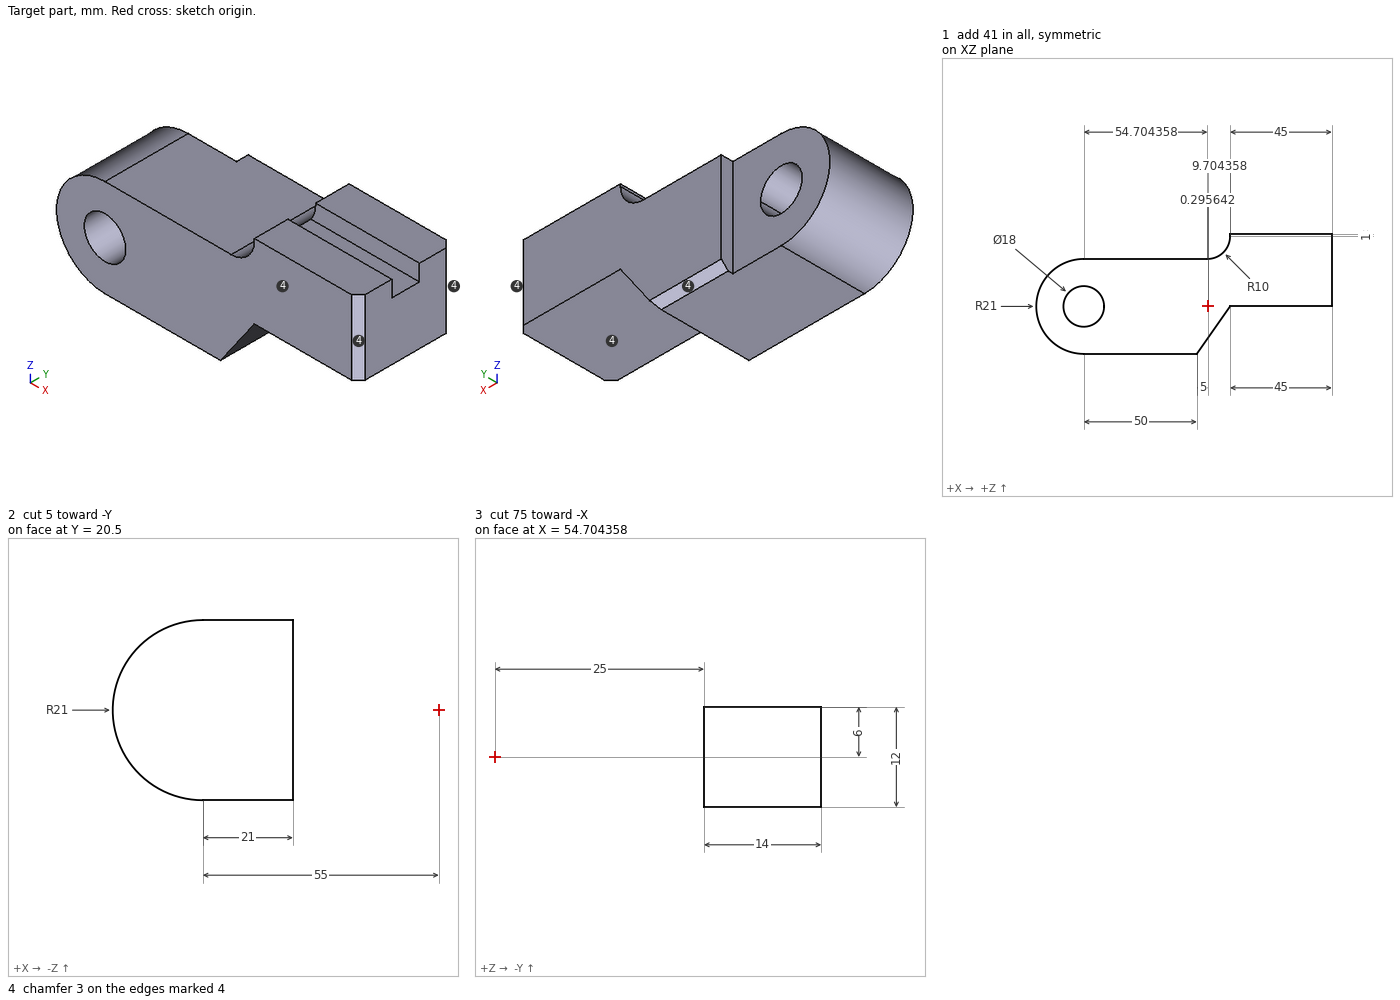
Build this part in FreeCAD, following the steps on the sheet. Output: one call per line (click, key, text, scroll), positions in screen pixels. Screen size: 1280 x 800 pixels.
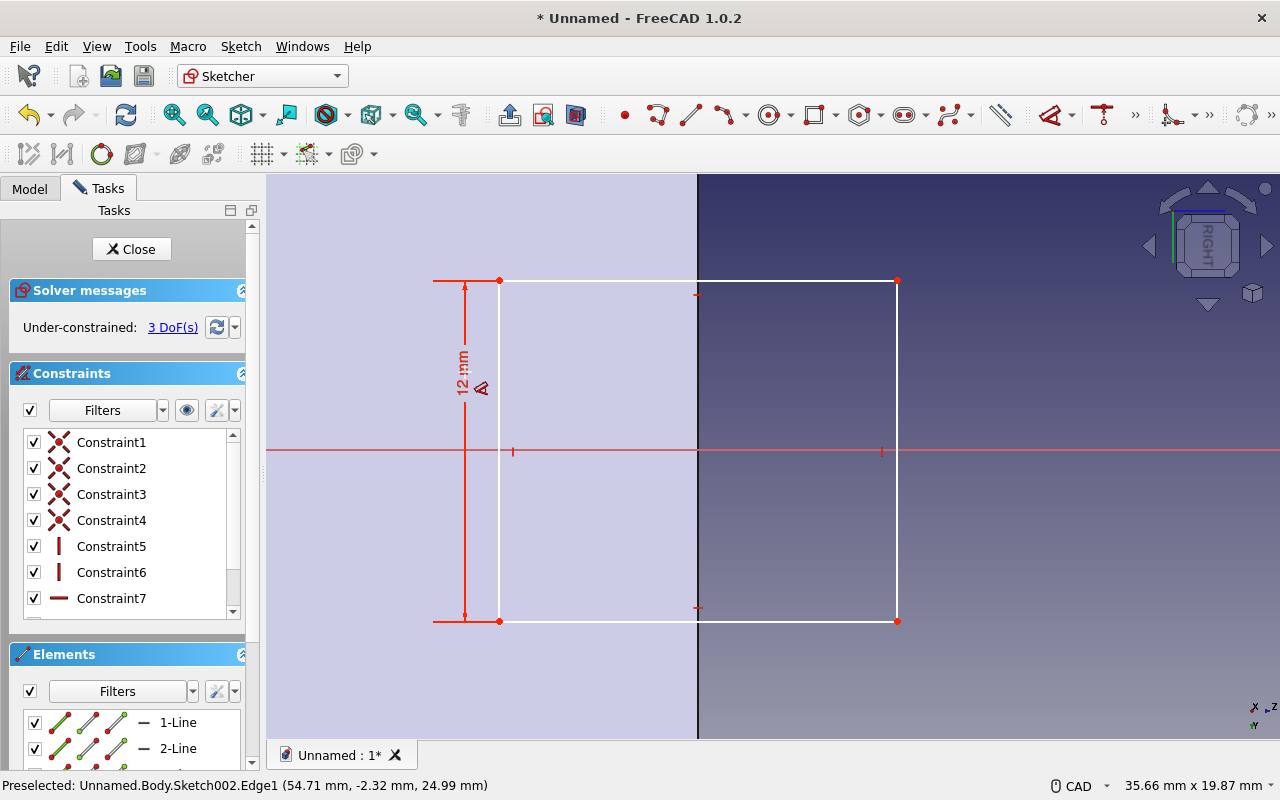
click(618, 622)
click(698, 656)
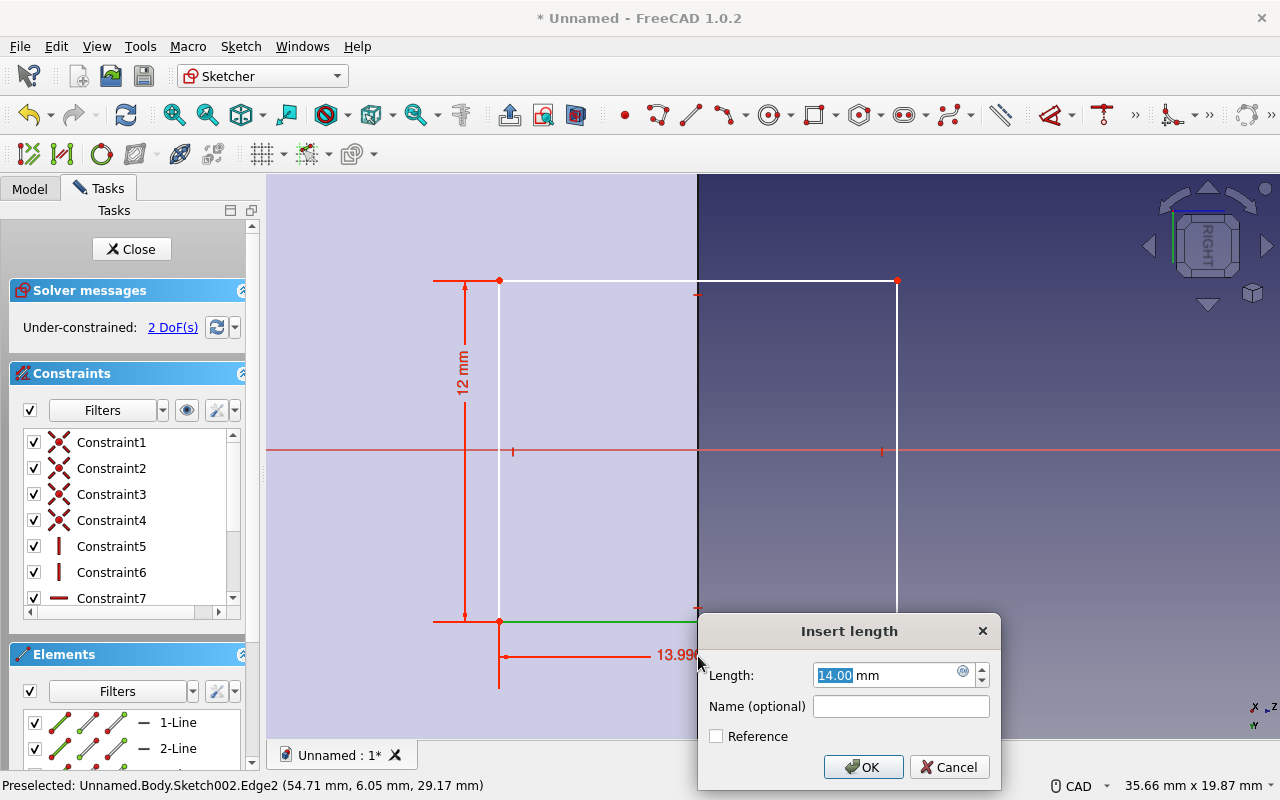
text(14)
key(Return)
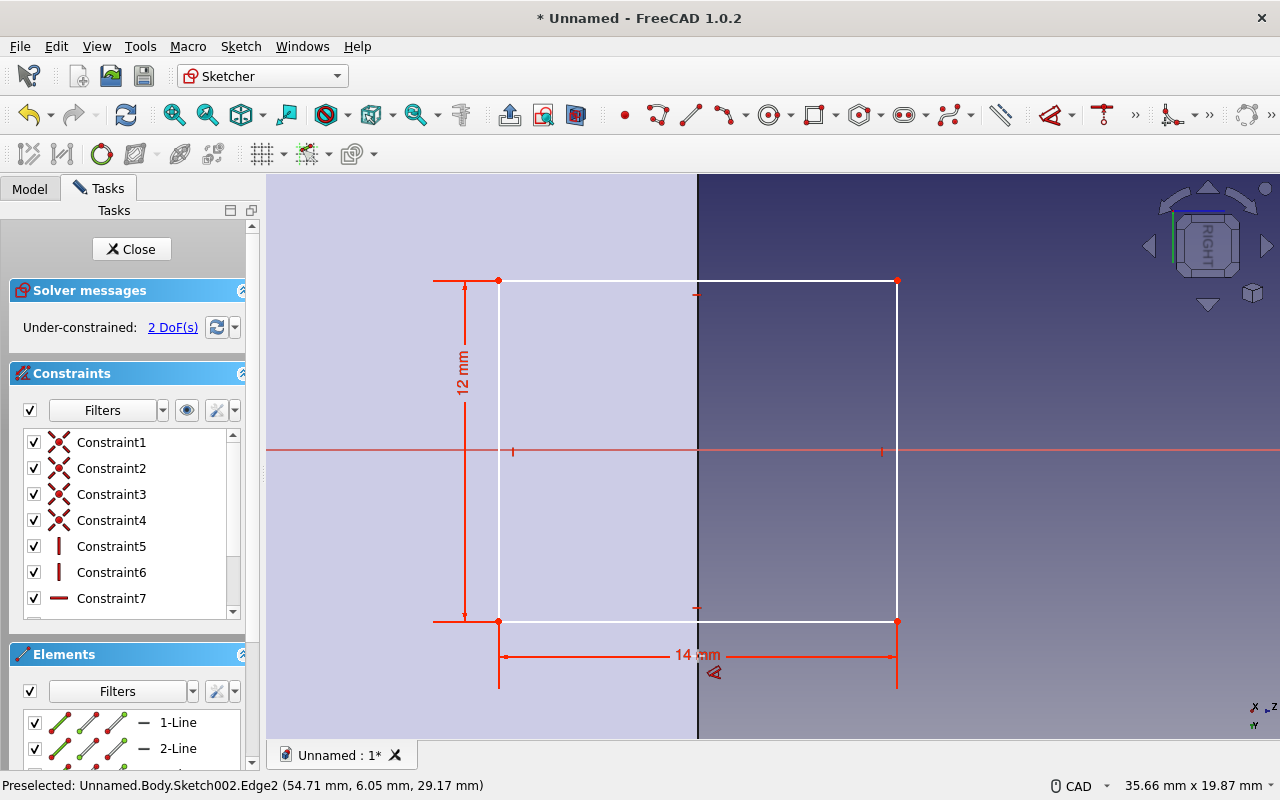
click(499, 281)
click(533, 326)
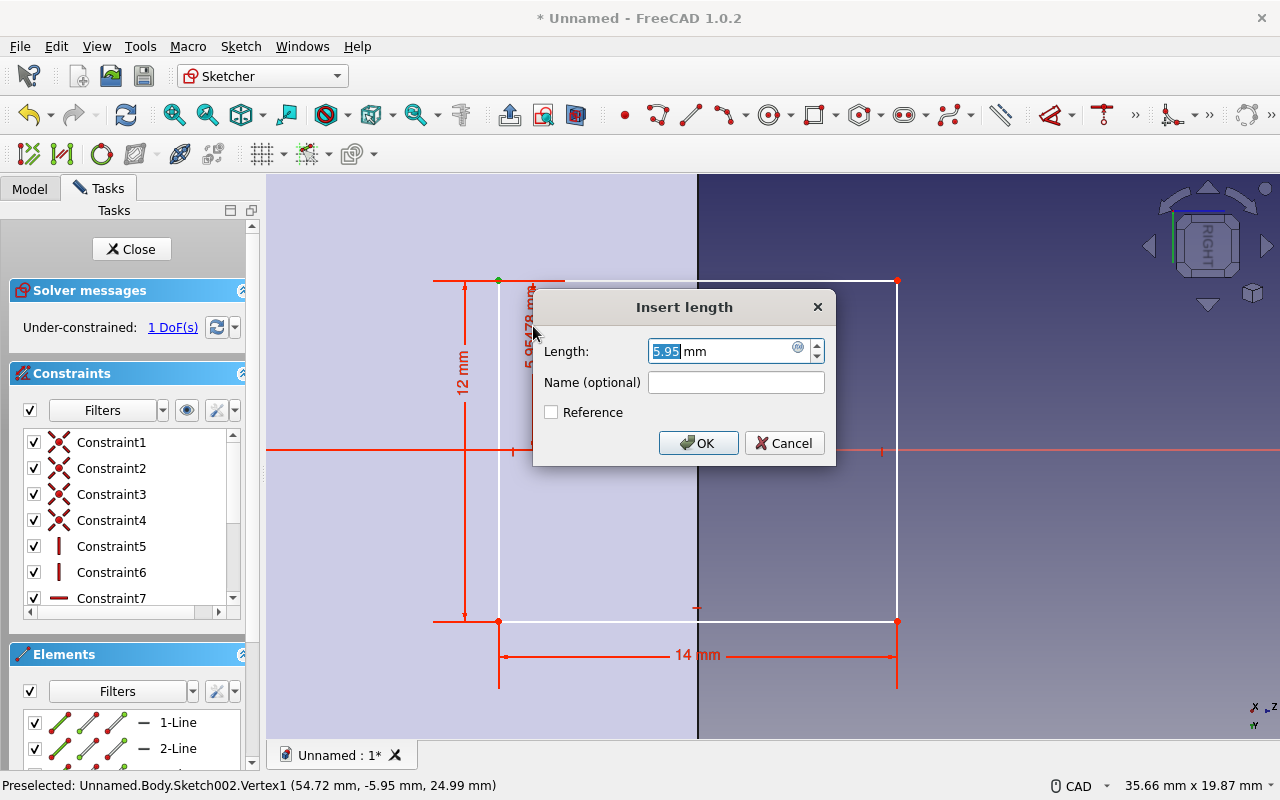
text(6)
key(Return)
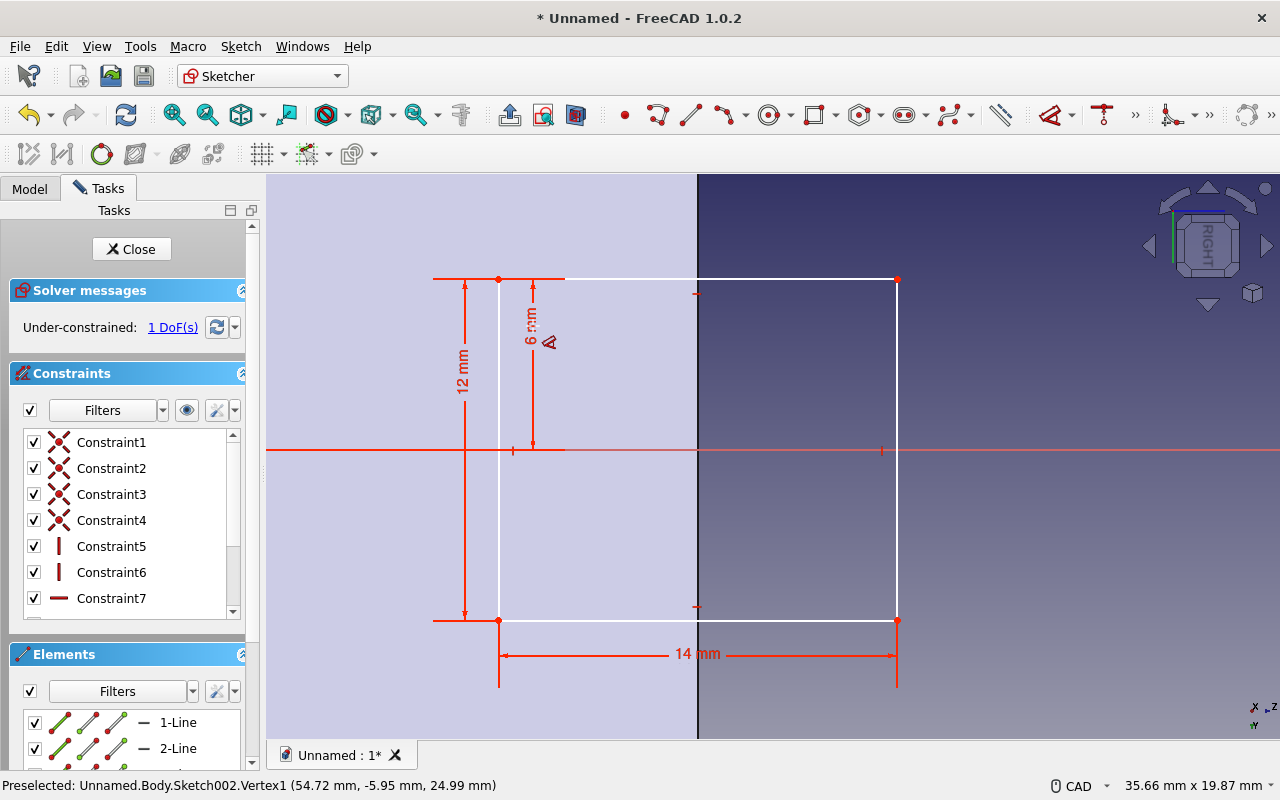
click(499, 279)
click(396, 245)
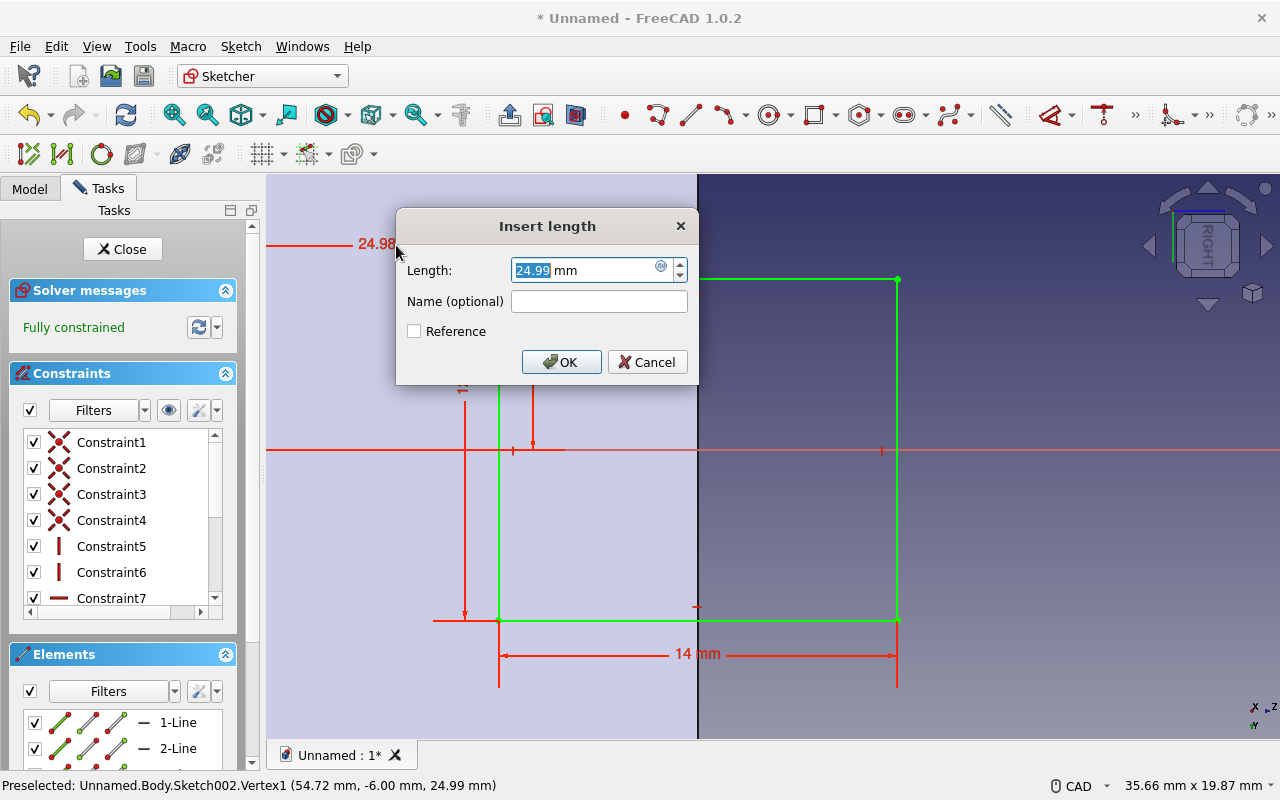
text(25)
key(Return)
key(Escape)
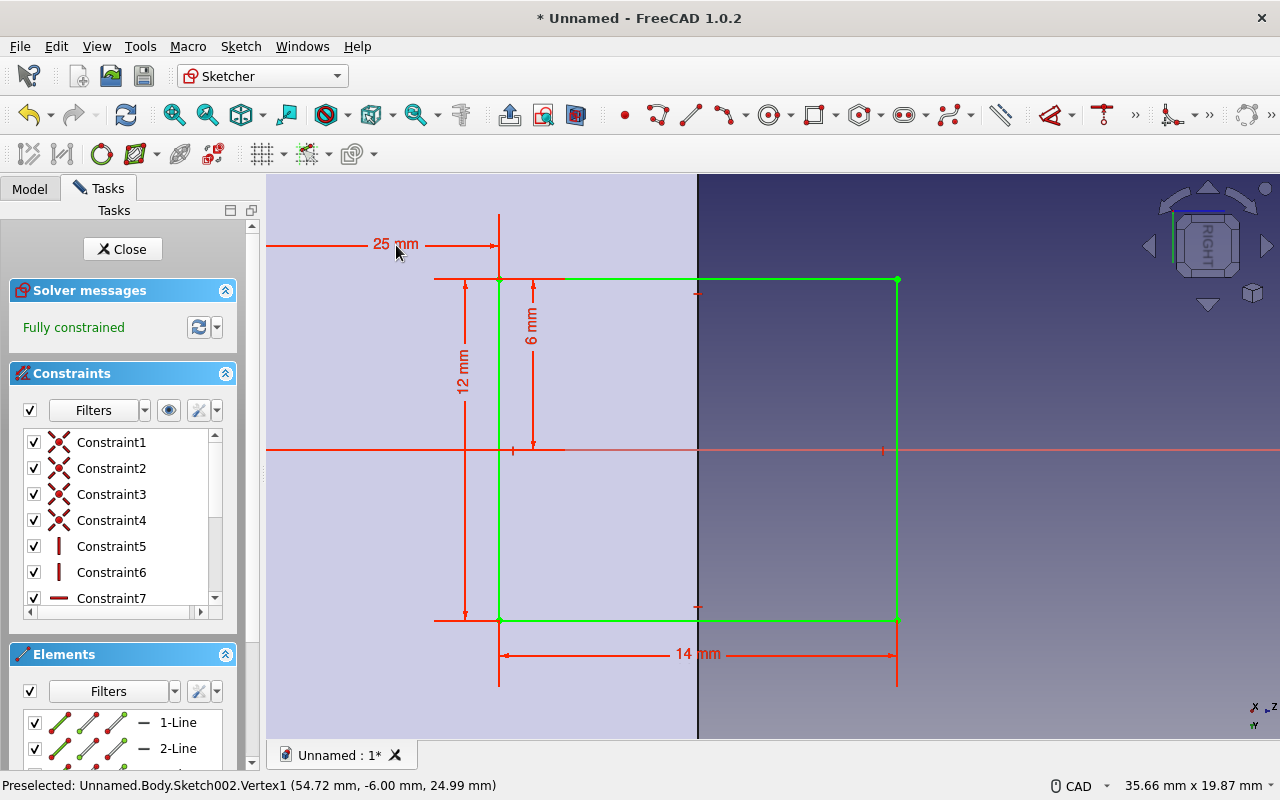
click(123, 249)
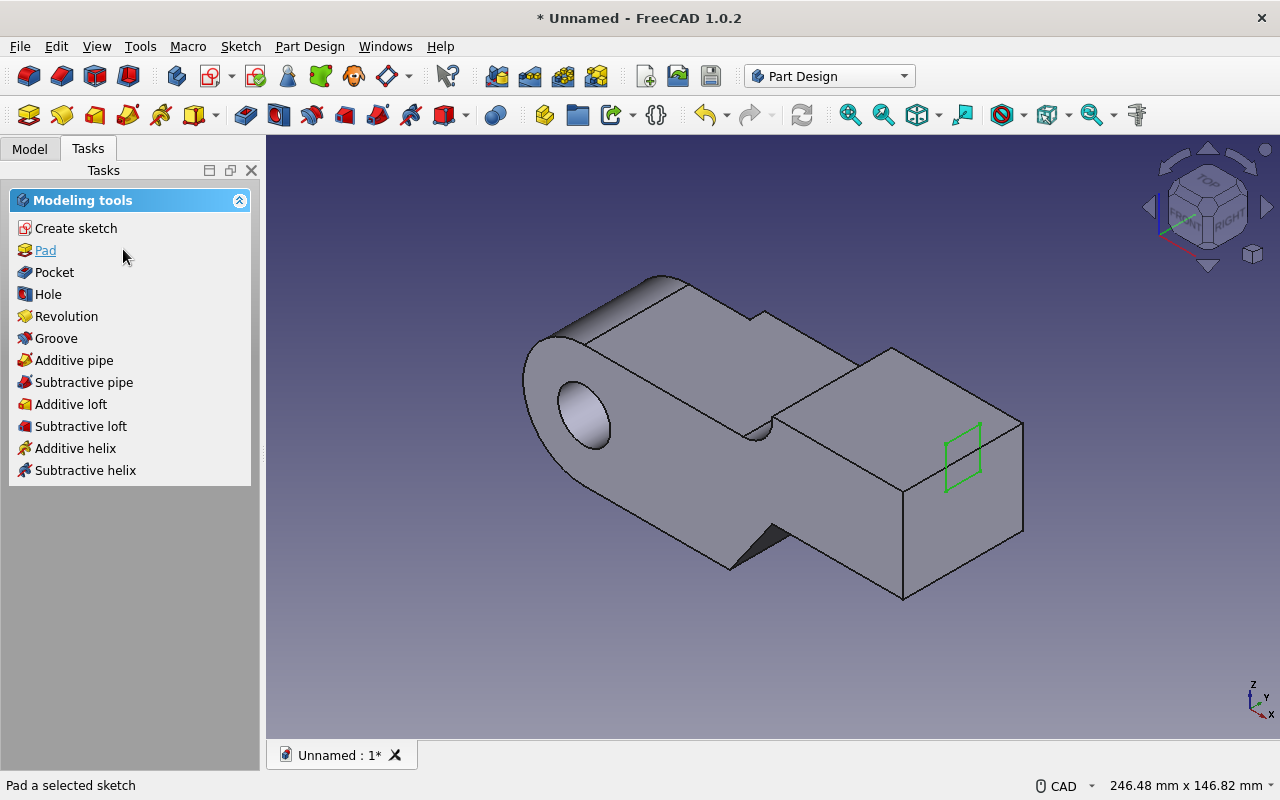
click(246, 116)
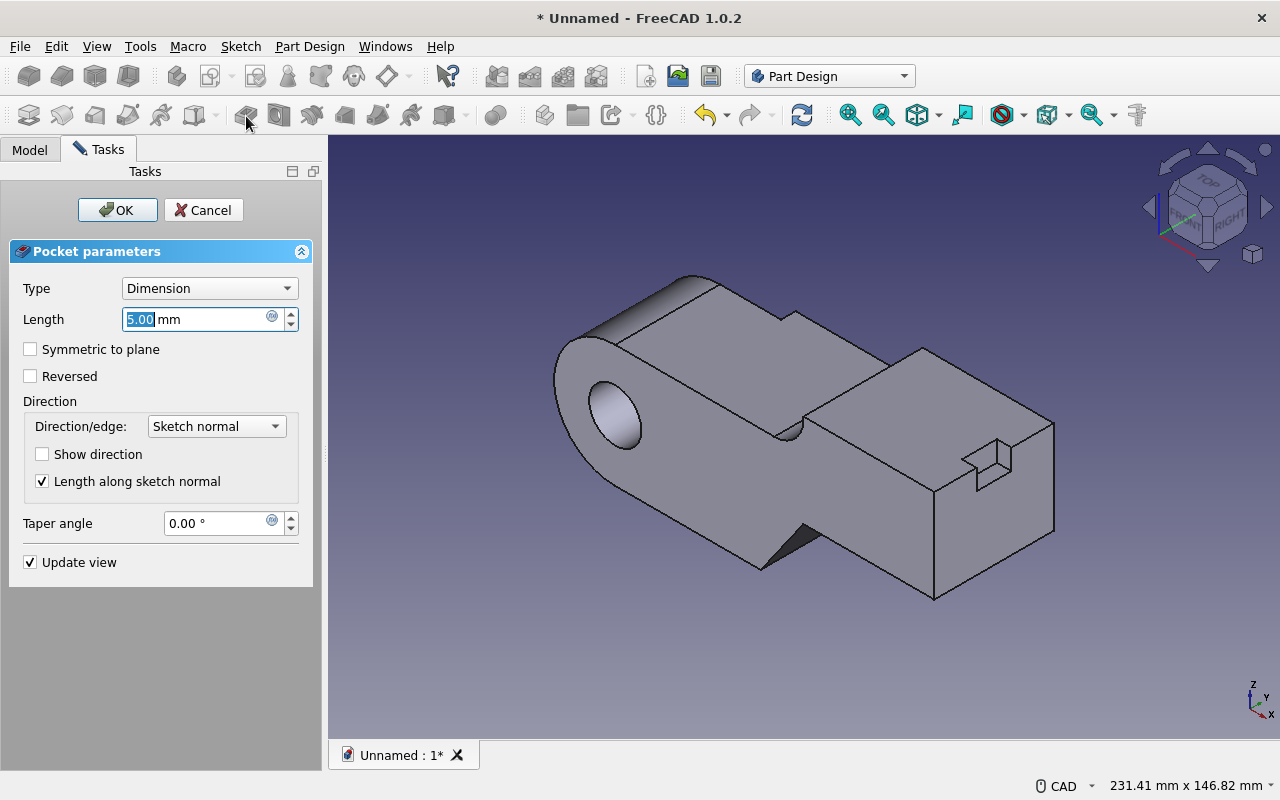
text(75)
key(Tab)